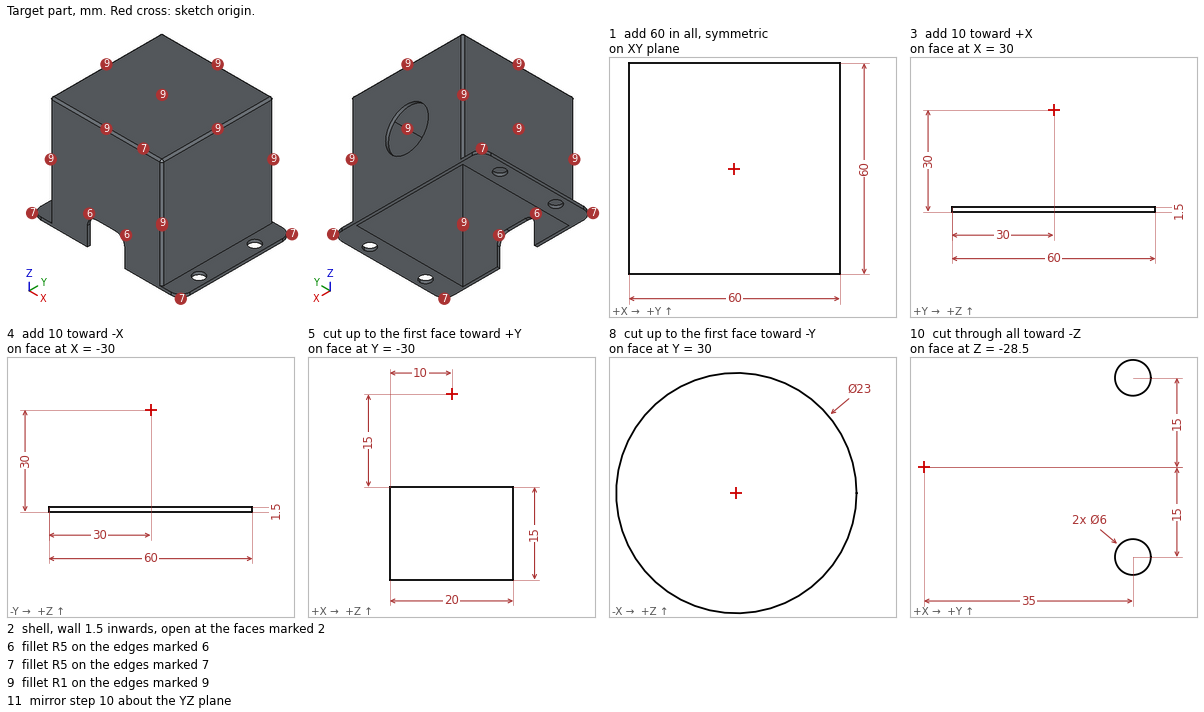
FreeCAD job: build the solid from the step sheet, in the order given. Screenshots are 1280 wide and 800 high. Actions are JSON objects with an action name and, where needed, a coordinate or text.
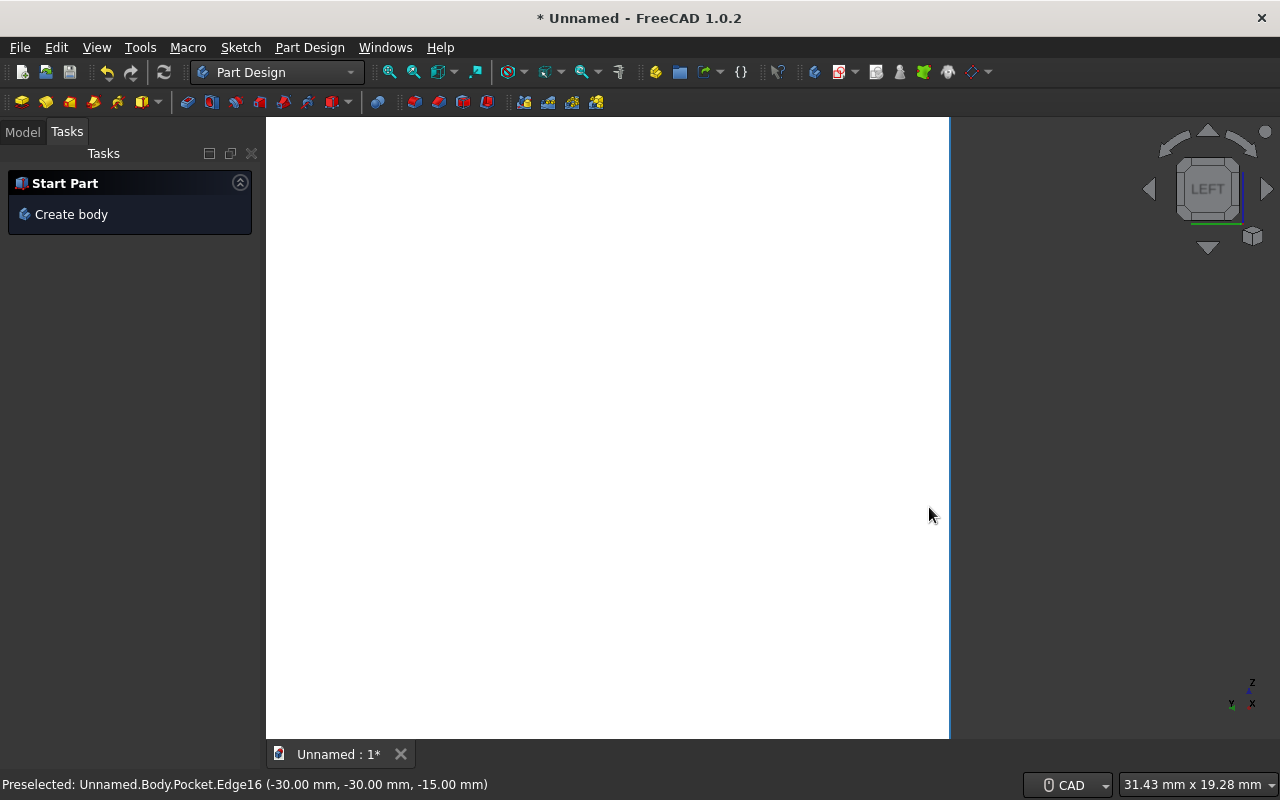
{"action": "left_click", "coordinate": [390, 72]}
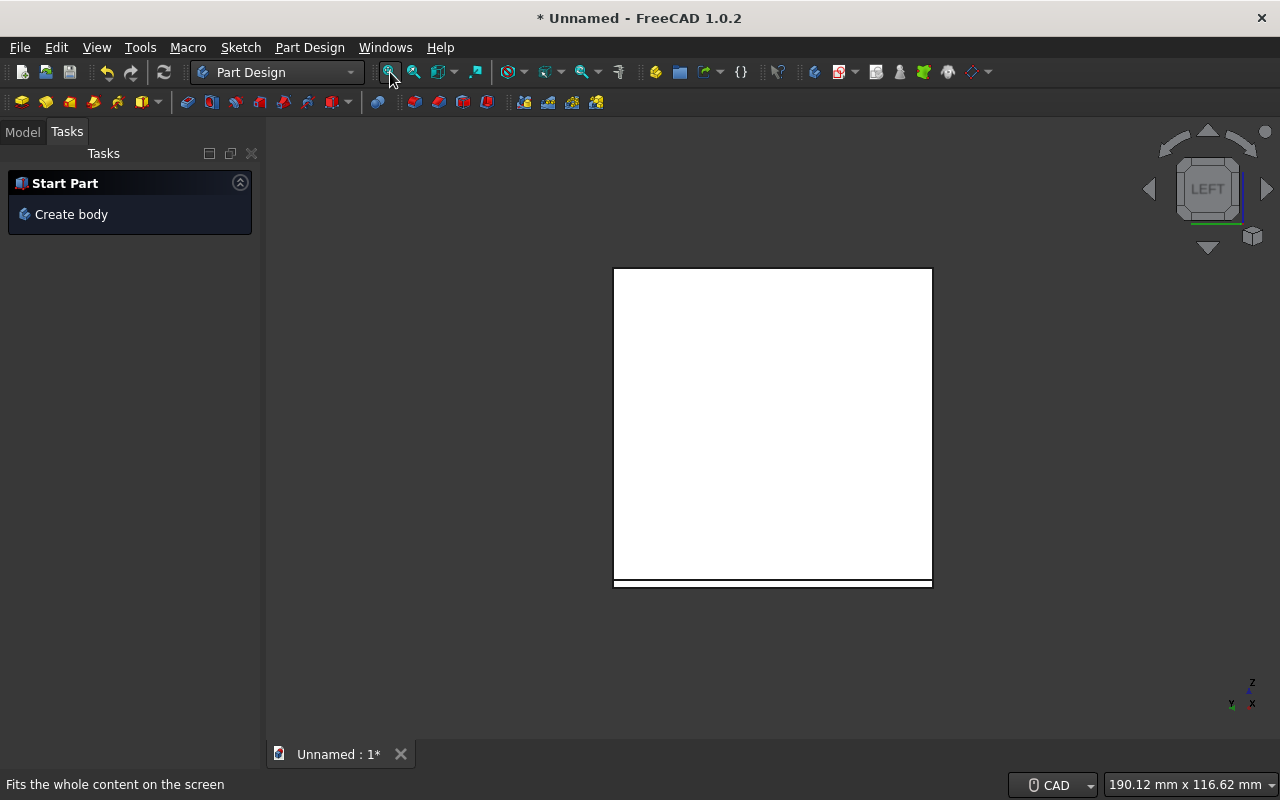
{"action": "key", "text": "v 3"}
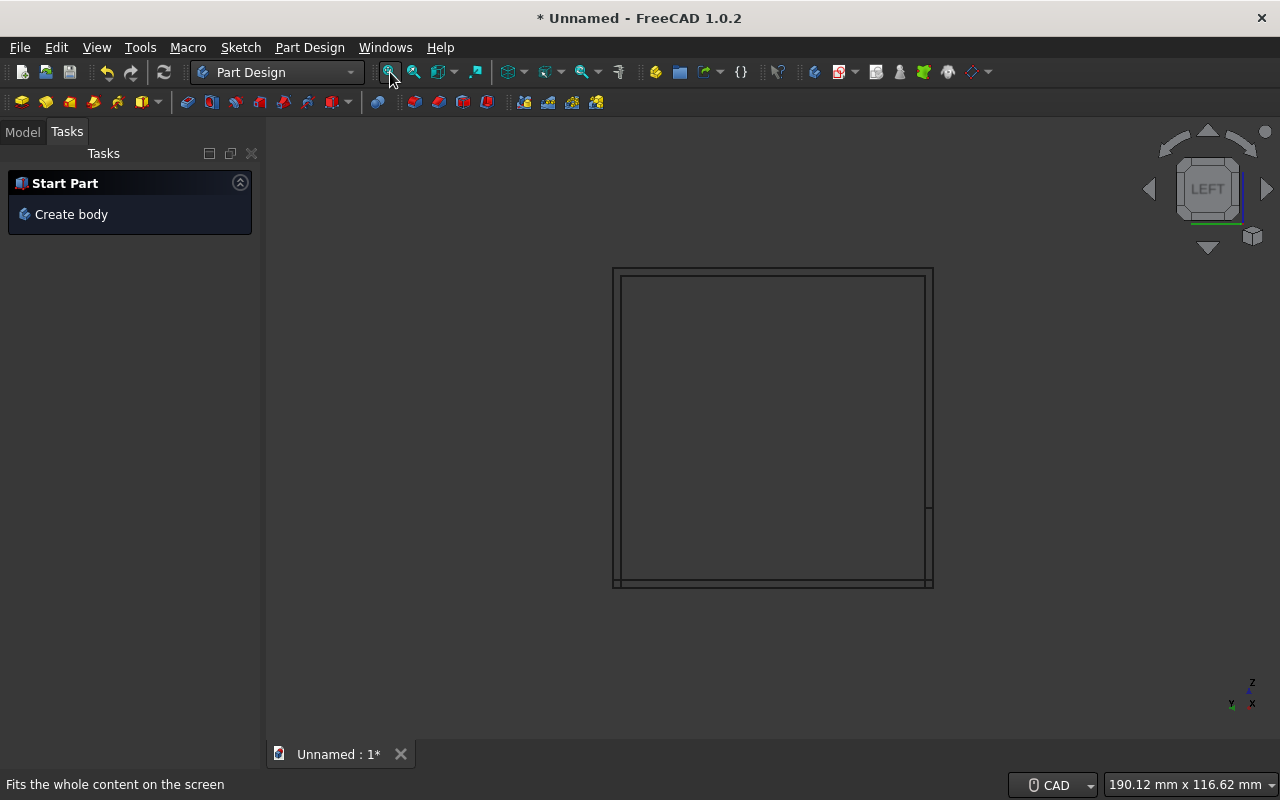
{"action": "key", "text": "0"}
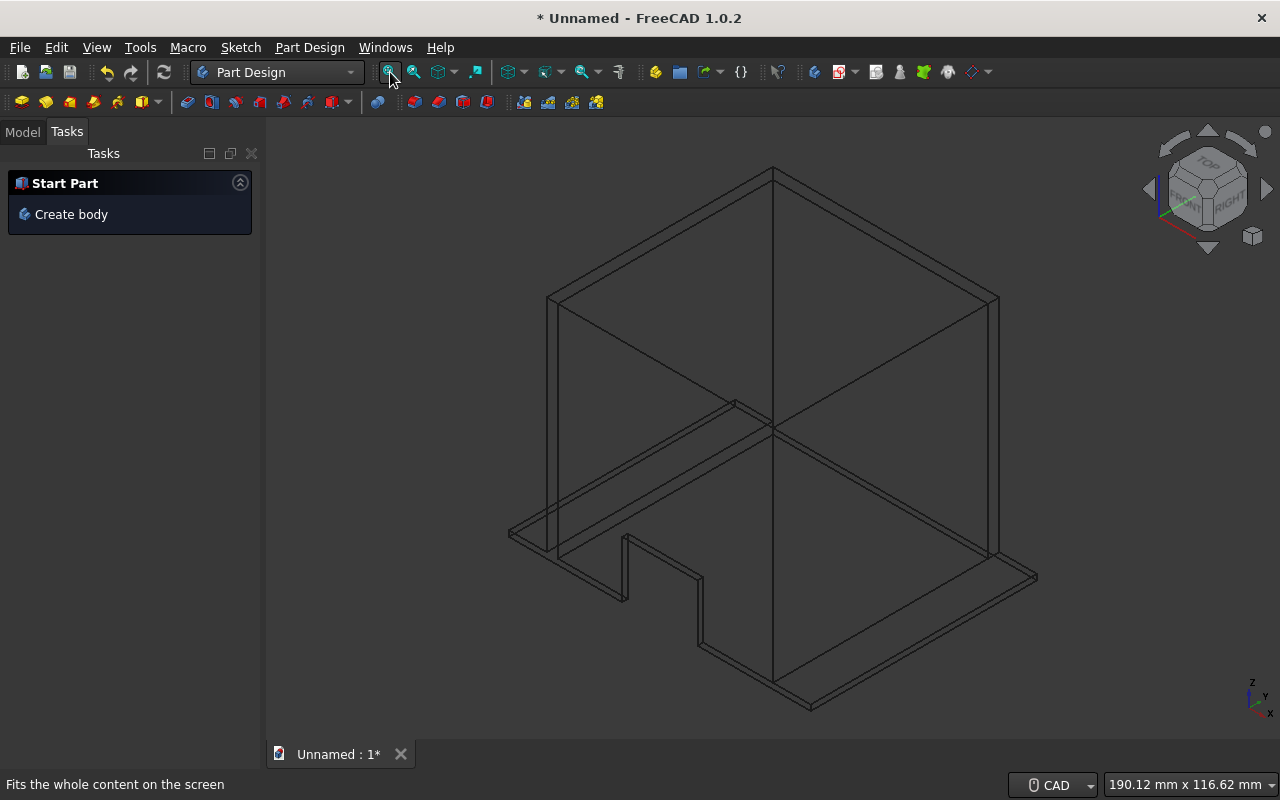
{"action": "scroll", "coordinate": [700, 578], "scroll_direction": "up", "scroll_amount": 9}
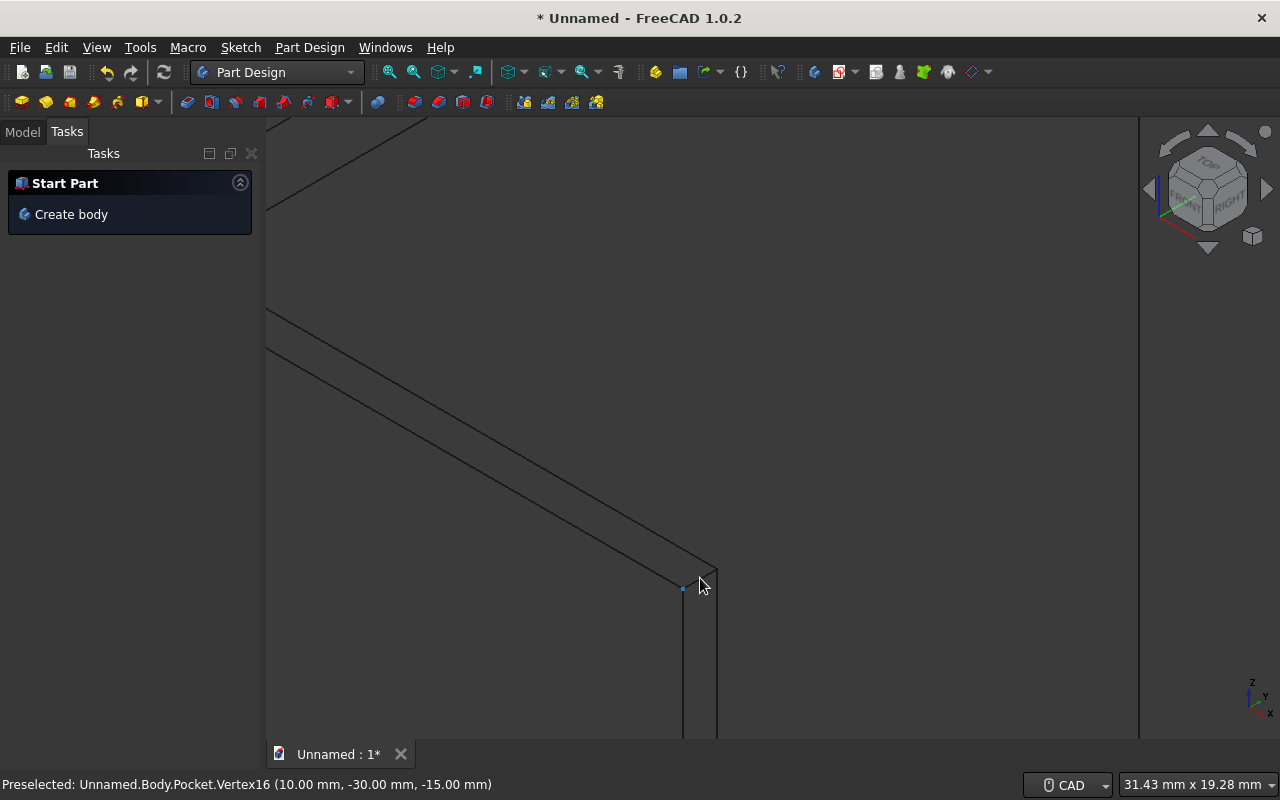
{"action": "left_click", "coordinate": [700, 578]}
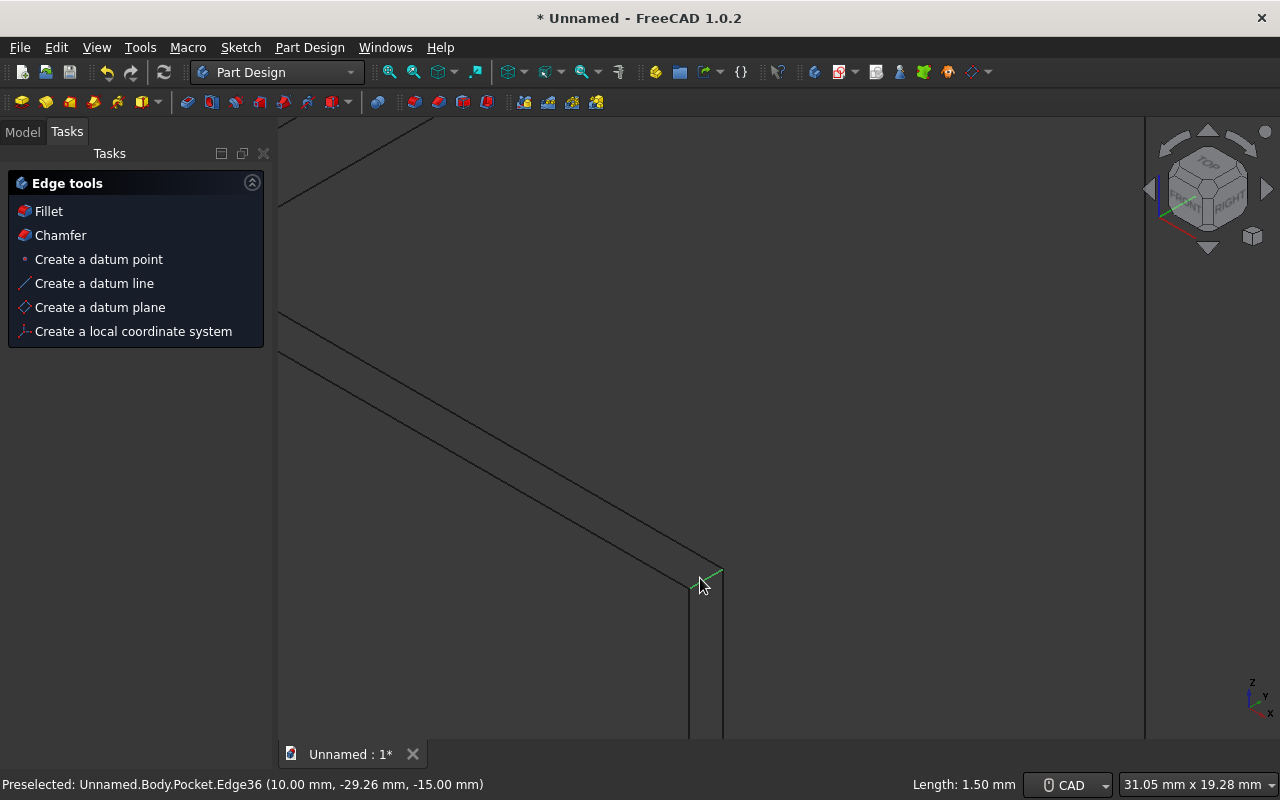
{"action": "key", "text": "v f"}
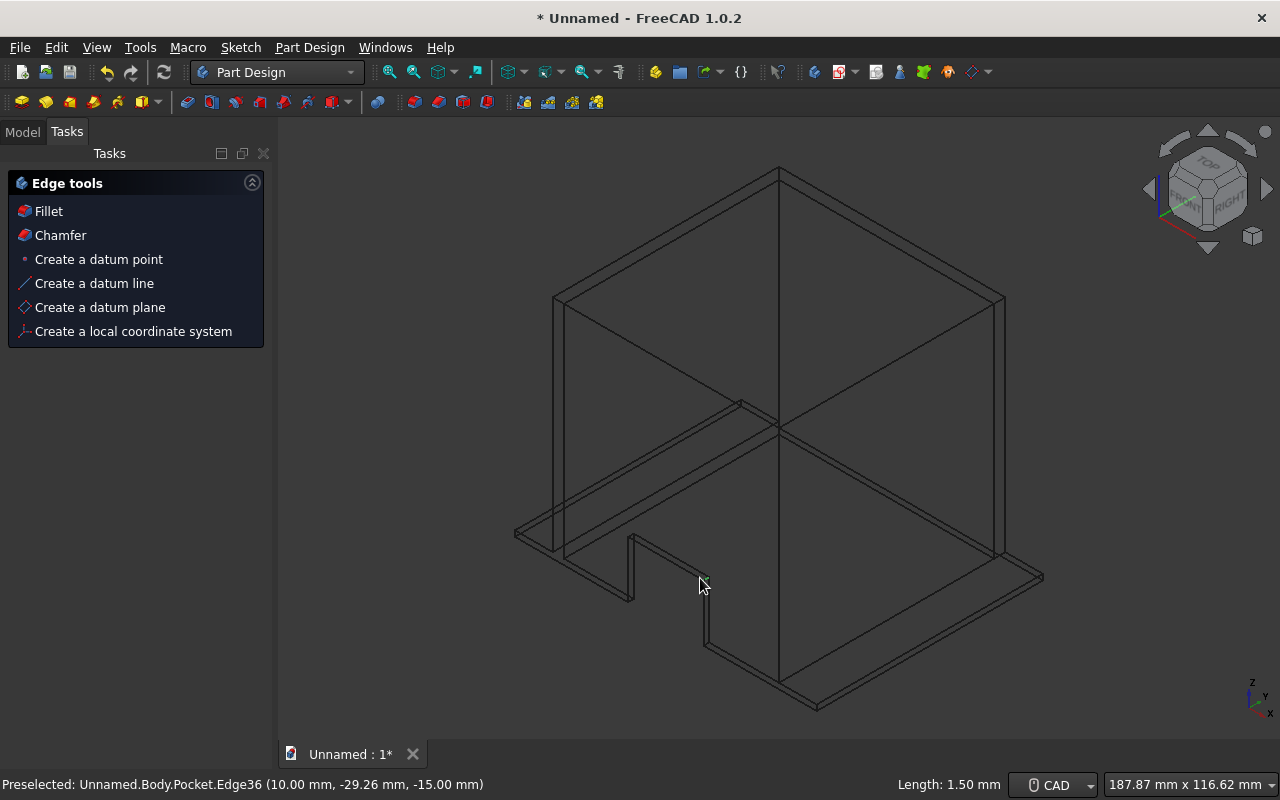
{"action": "key", "text": "2"}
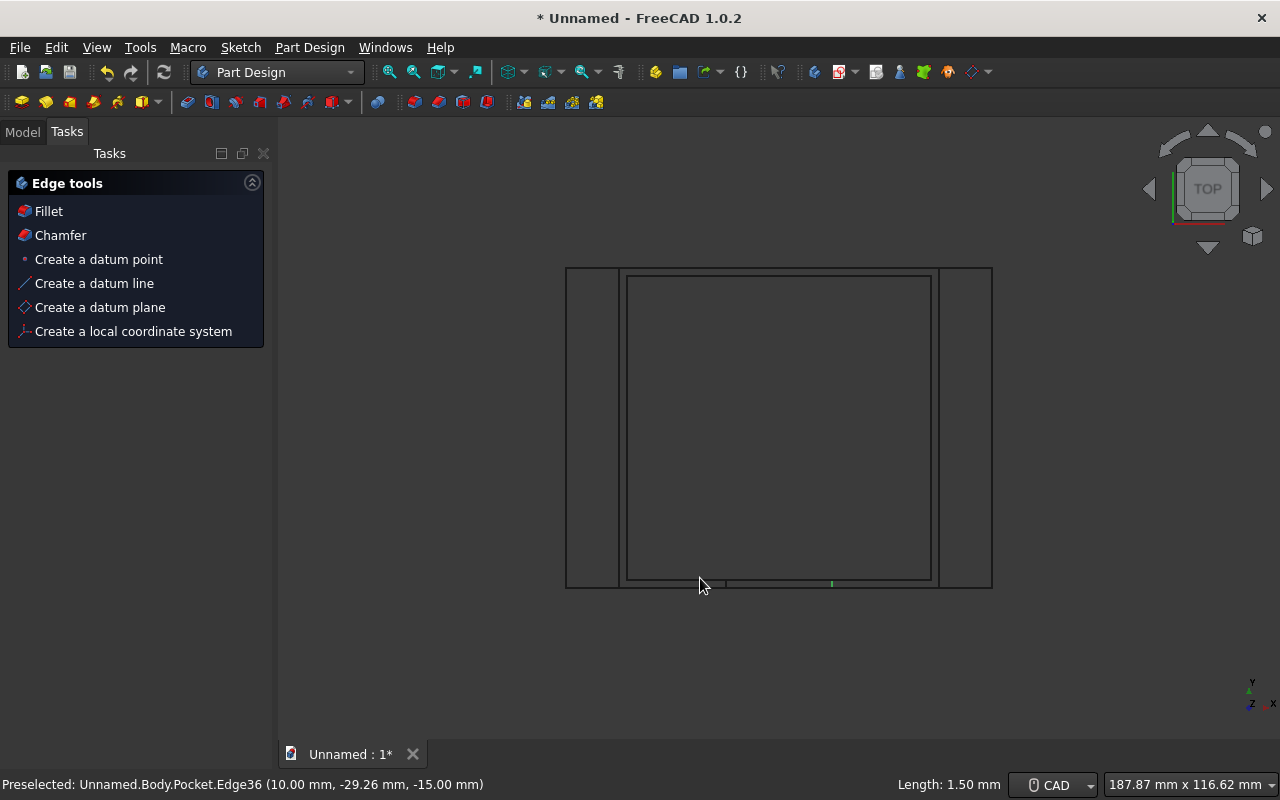
{"action": "scroll", "coordinate": [726, 583], "scroll_direction": "up", "scroll_amount": 9}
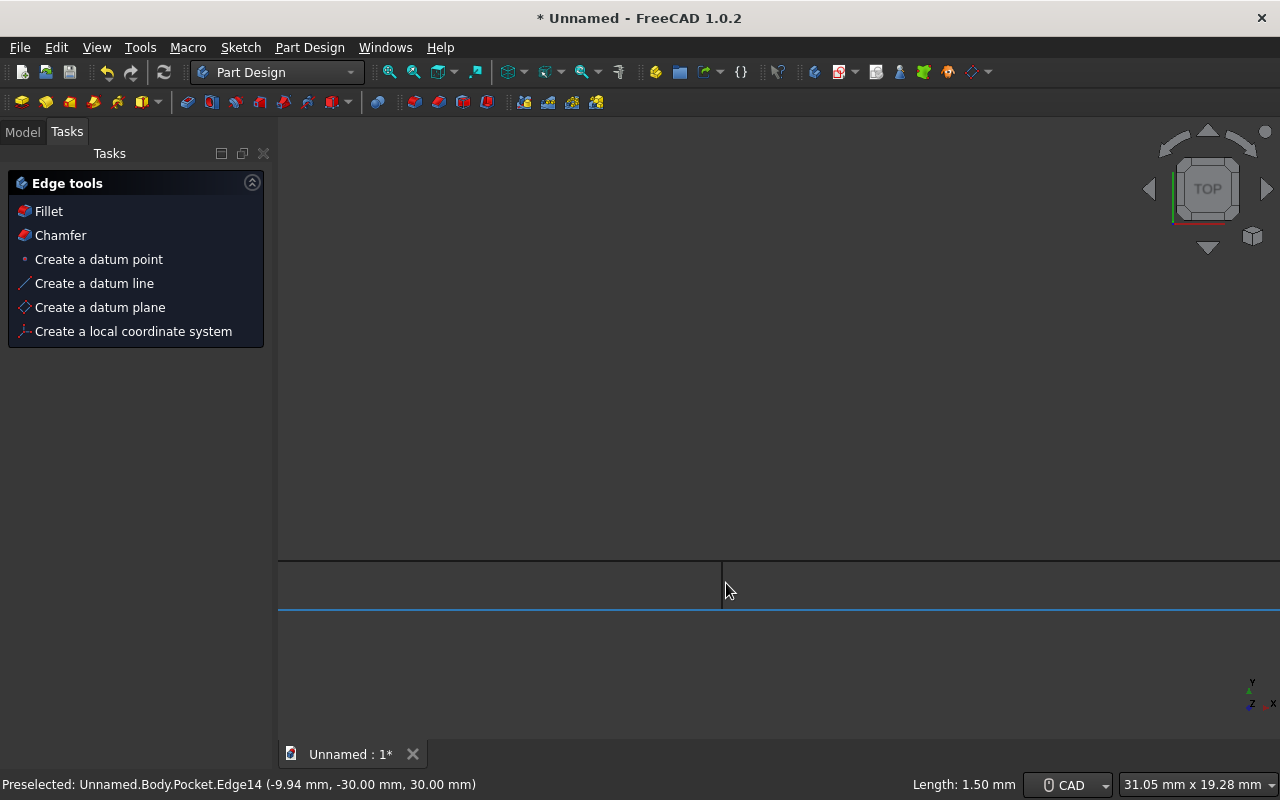
{"action": "left_click", "coordinate": [722, 584], "text": "ctrl"}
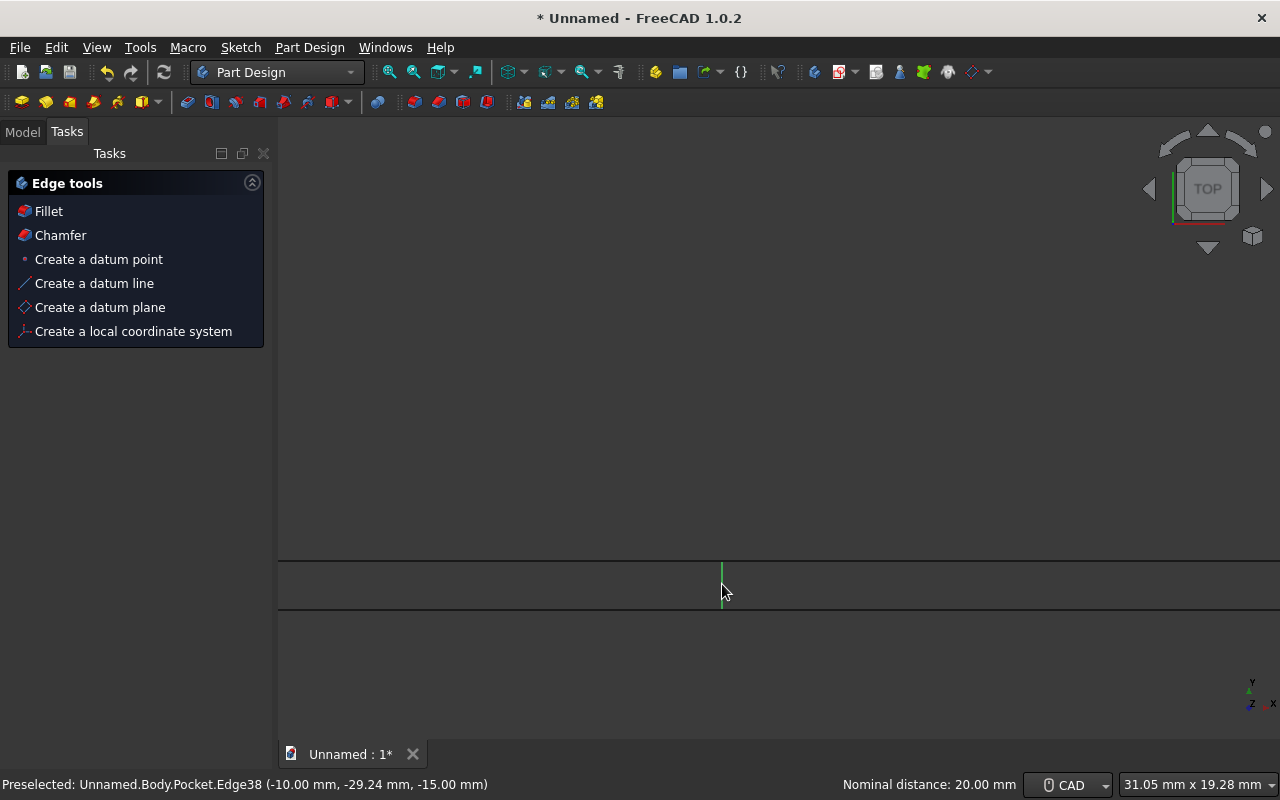
{"action": "key", "text": "v 1"}